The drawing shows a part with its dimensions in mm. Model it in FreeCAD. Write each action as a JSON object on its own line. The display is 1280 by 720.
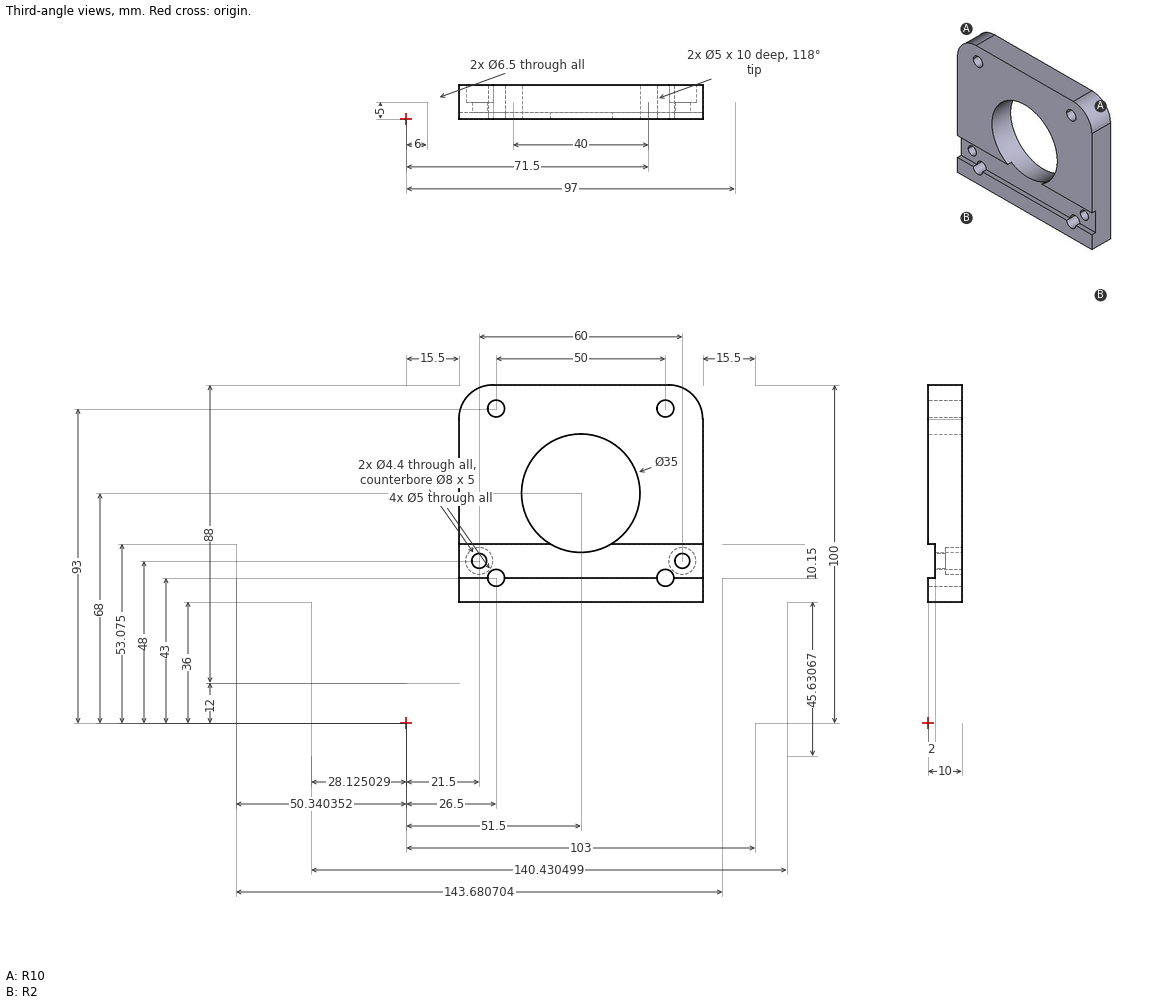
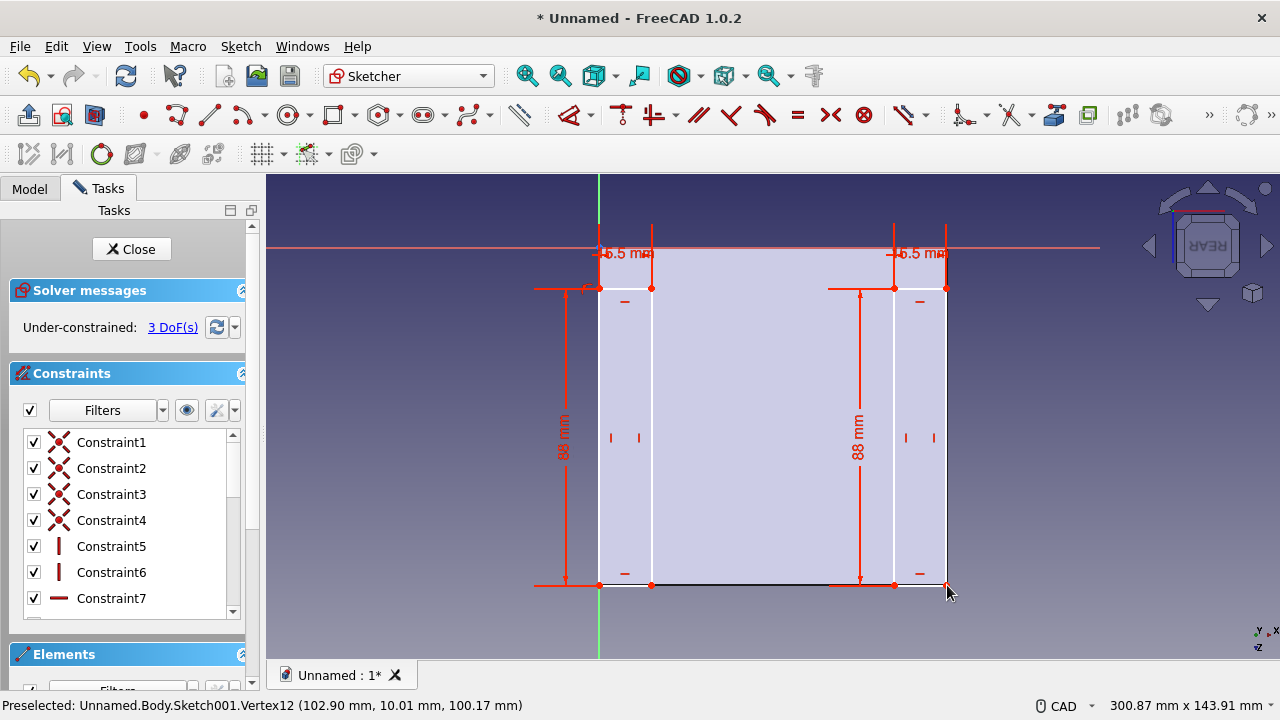
{"action": "left_click", "coordinate": [568, 116]}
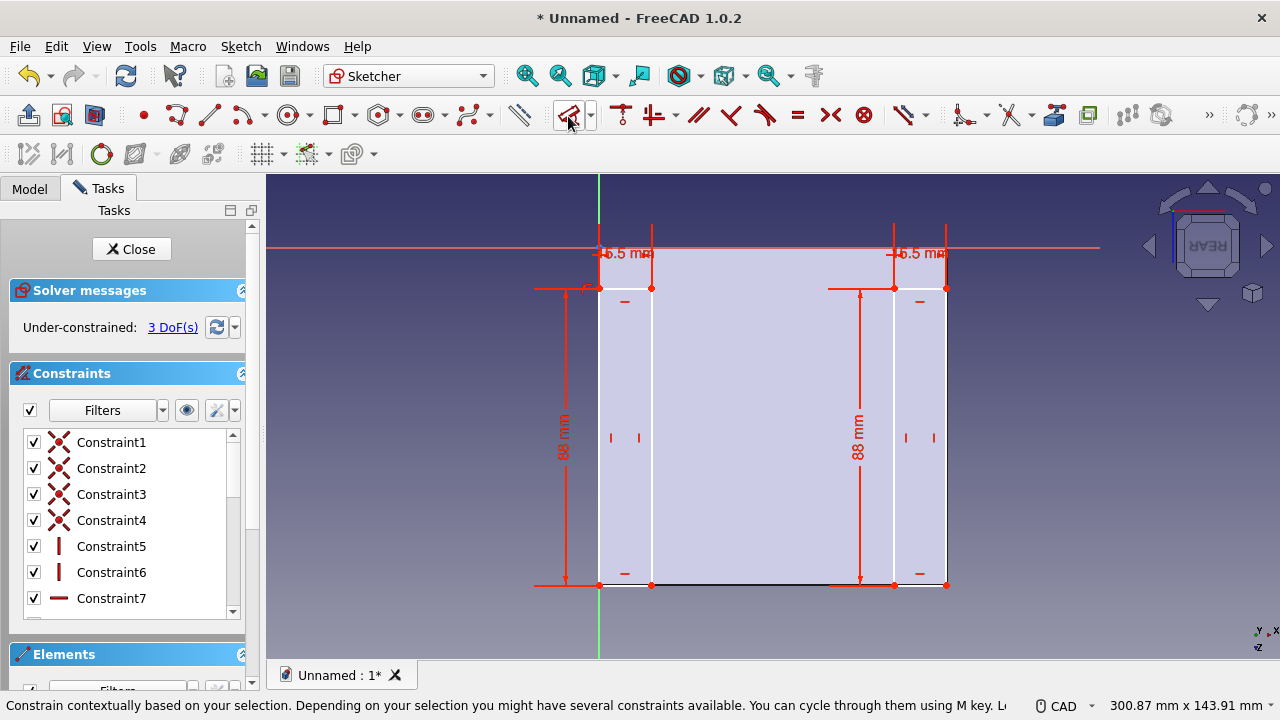
{"action": "left_click", "coordinate": [599, 289]}
{"action": "left_click", "coordinate": [565, 268]}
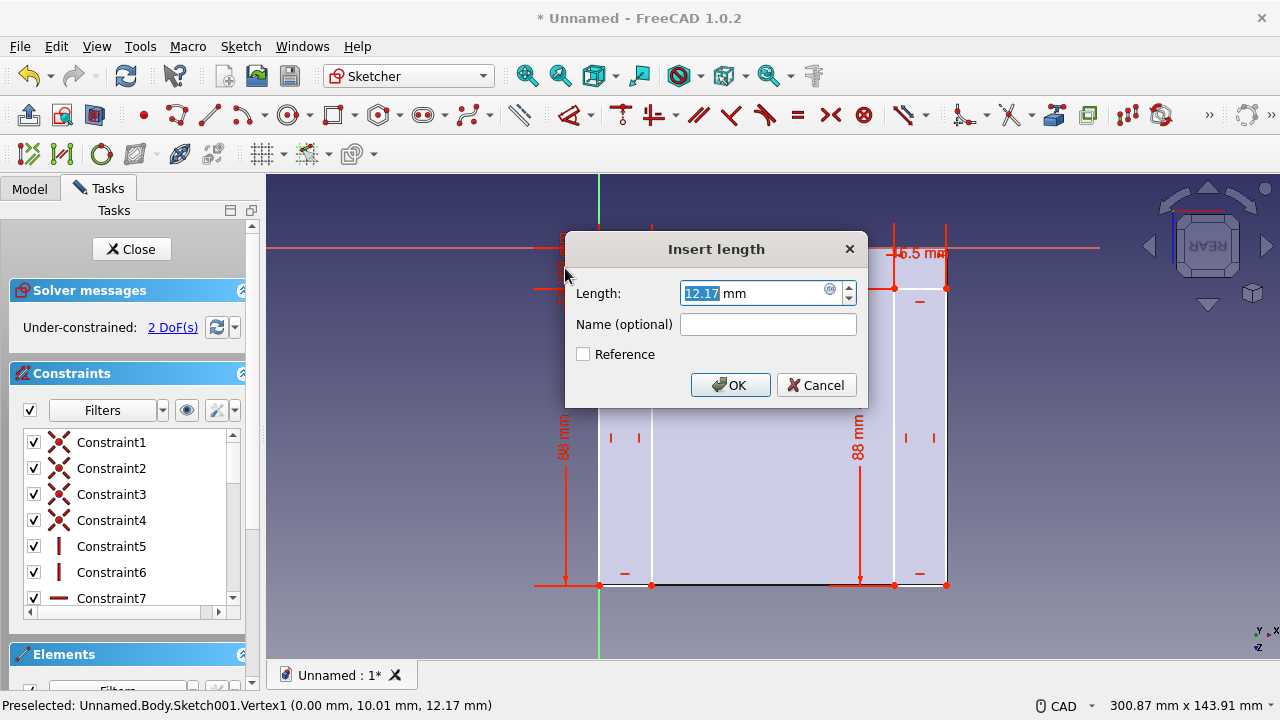
{"action": "type", "text": "12"}
{"action": "key", "text": "Return"}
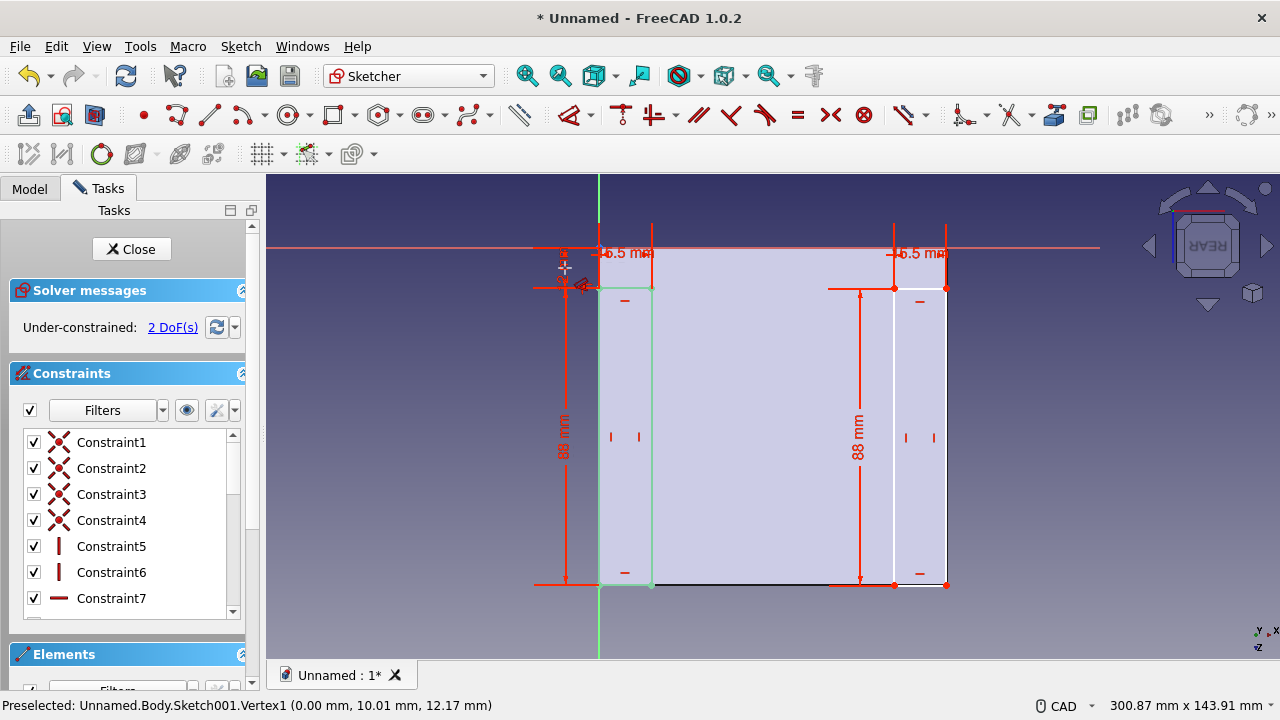
{"action": "left_click", "coordinate": [894, 289]}
{"action": "left_click", "coordinate": [928, 268]}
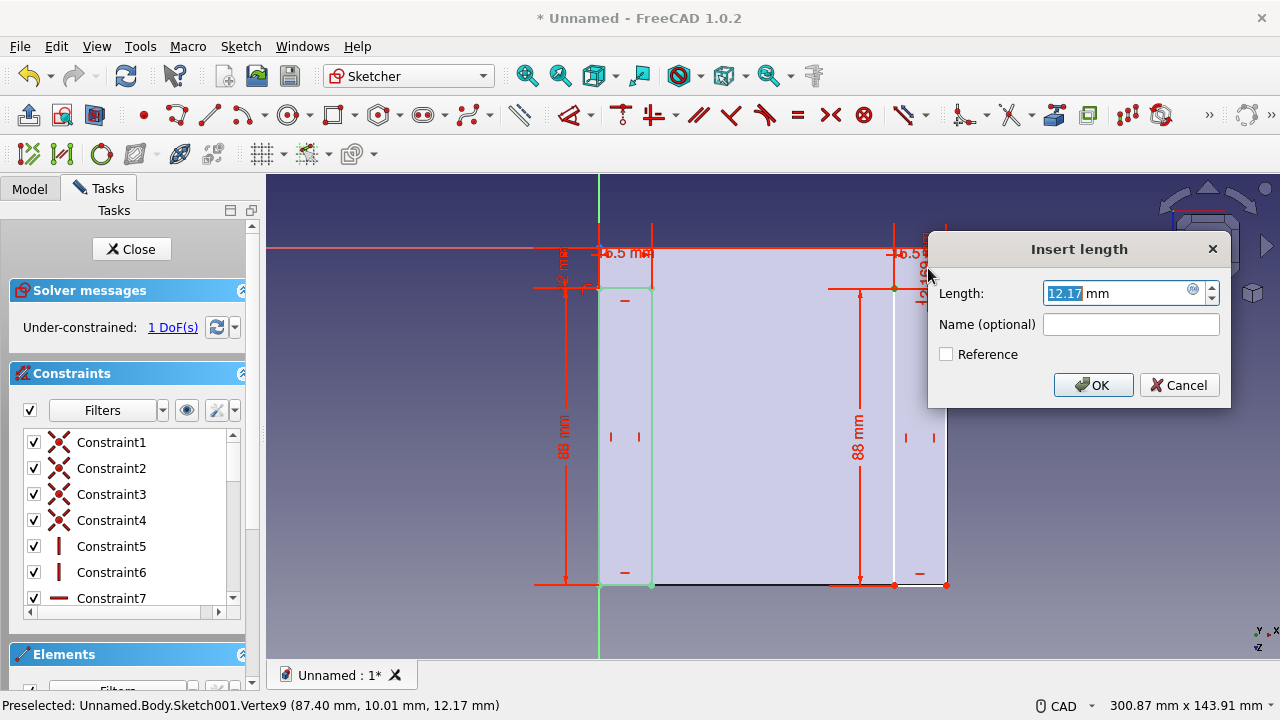
{"action": "type", "text": "12"}
{"action": "key", "text": "Return"}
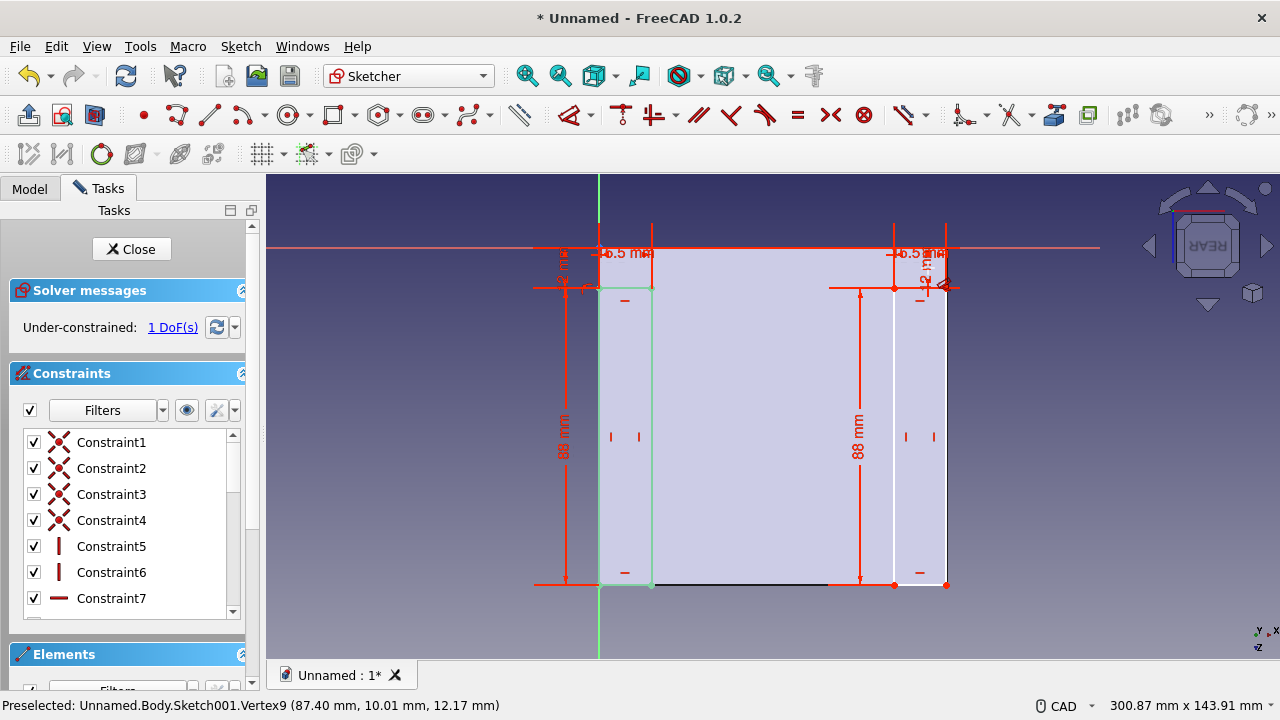
{"action": "left_click", "coordinate": [946, 585]}
{"action": "left_click", "coordinate": [773, 619]}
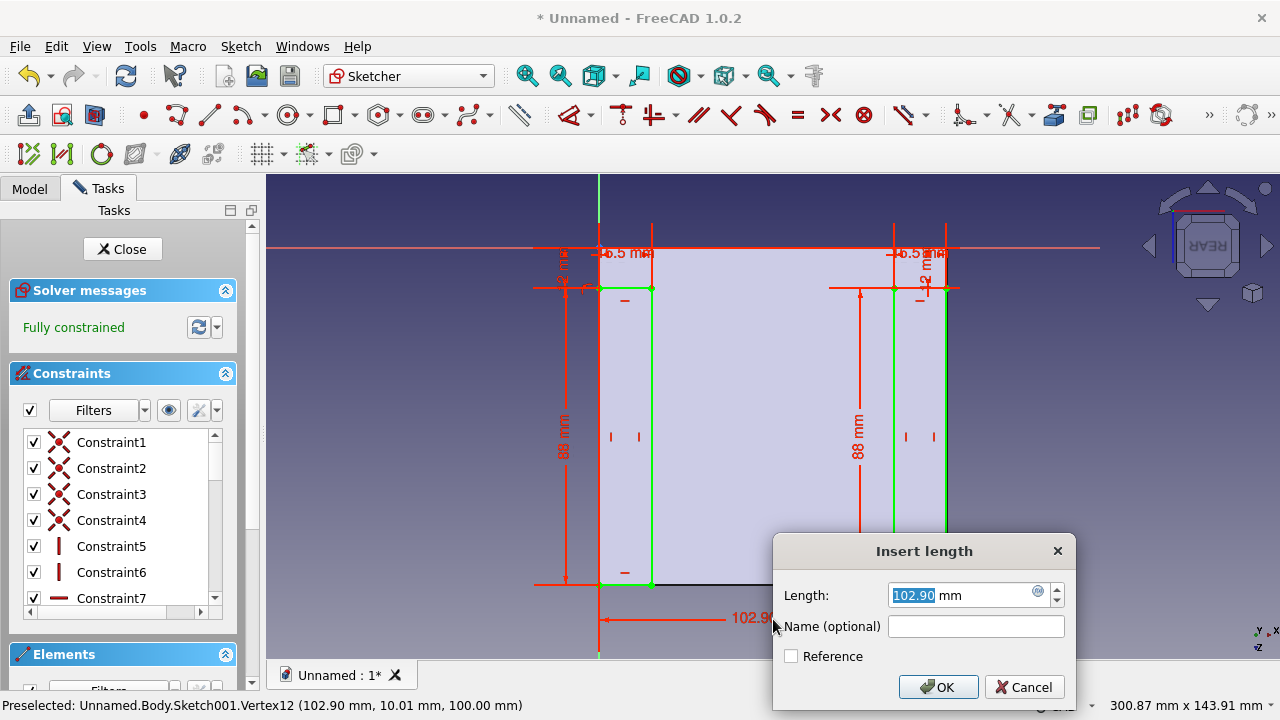
{"action": "type", "text": "103"}
{"action": "key", "text": "Return"}
{"action": "key", "text": "Escape"}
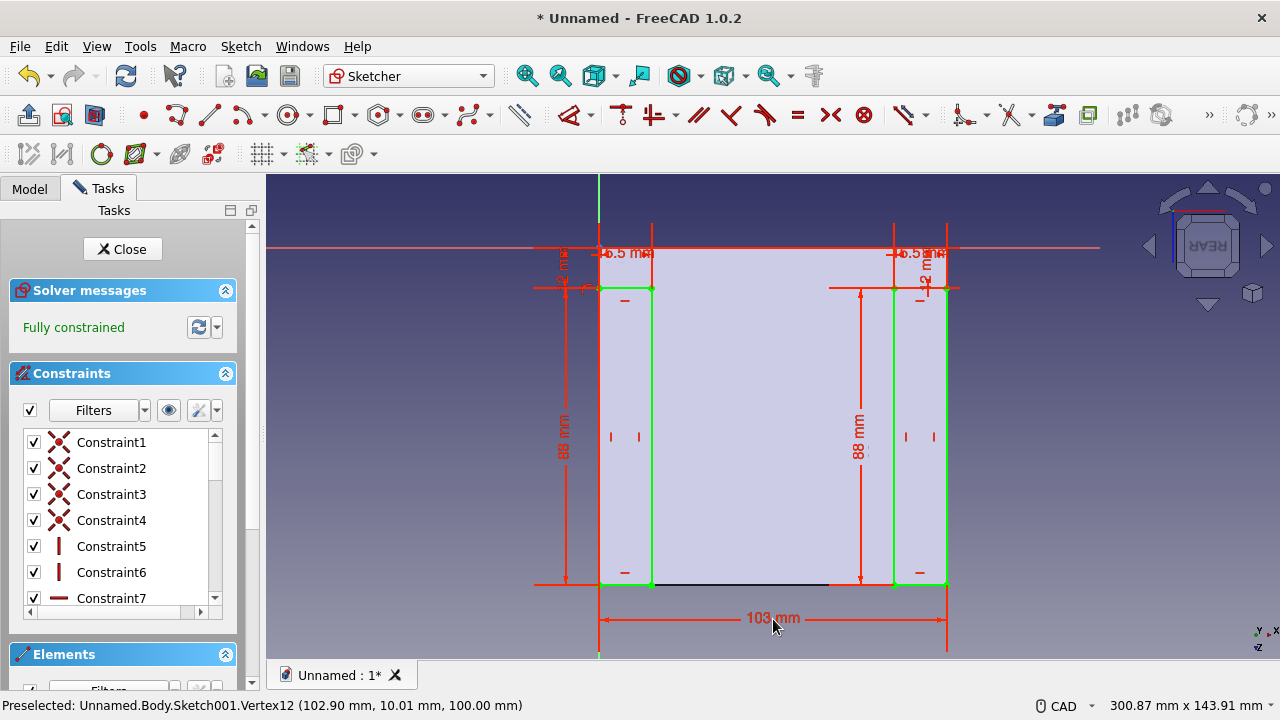
{"action": "left_click", "coordinate": [123, 249]}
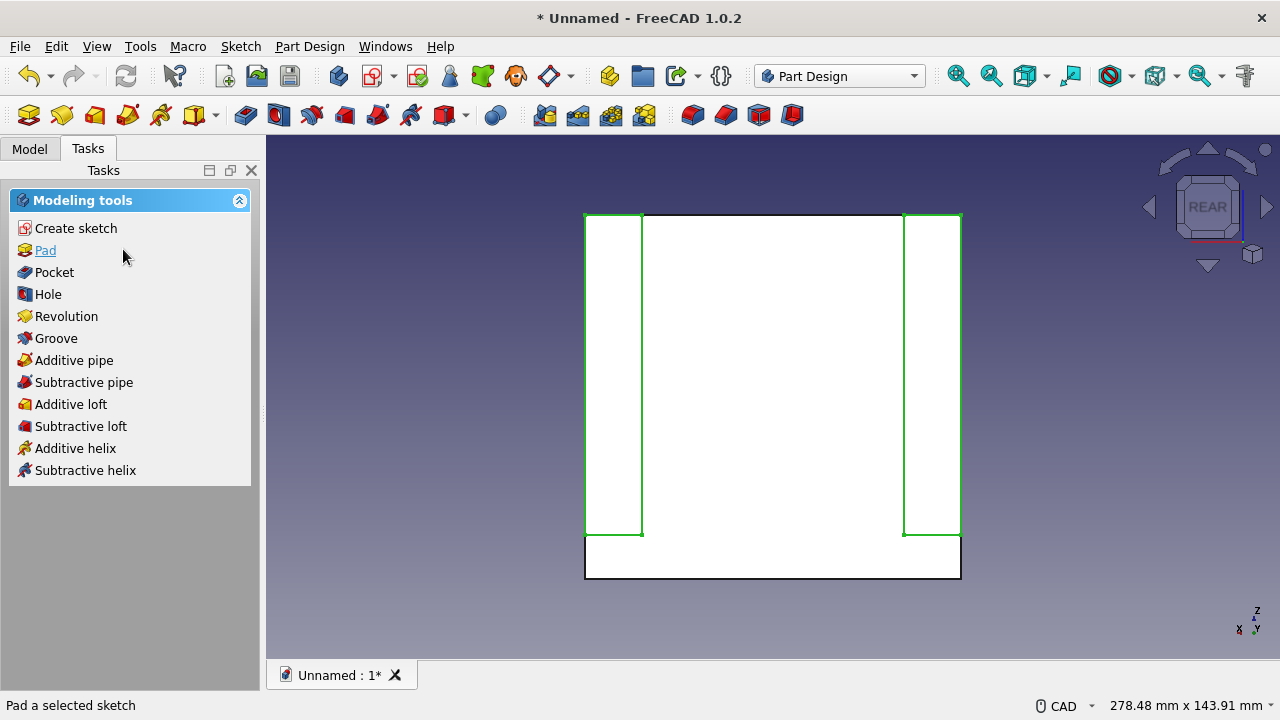
{"action": "left_click", "coordinate": [246, 116]}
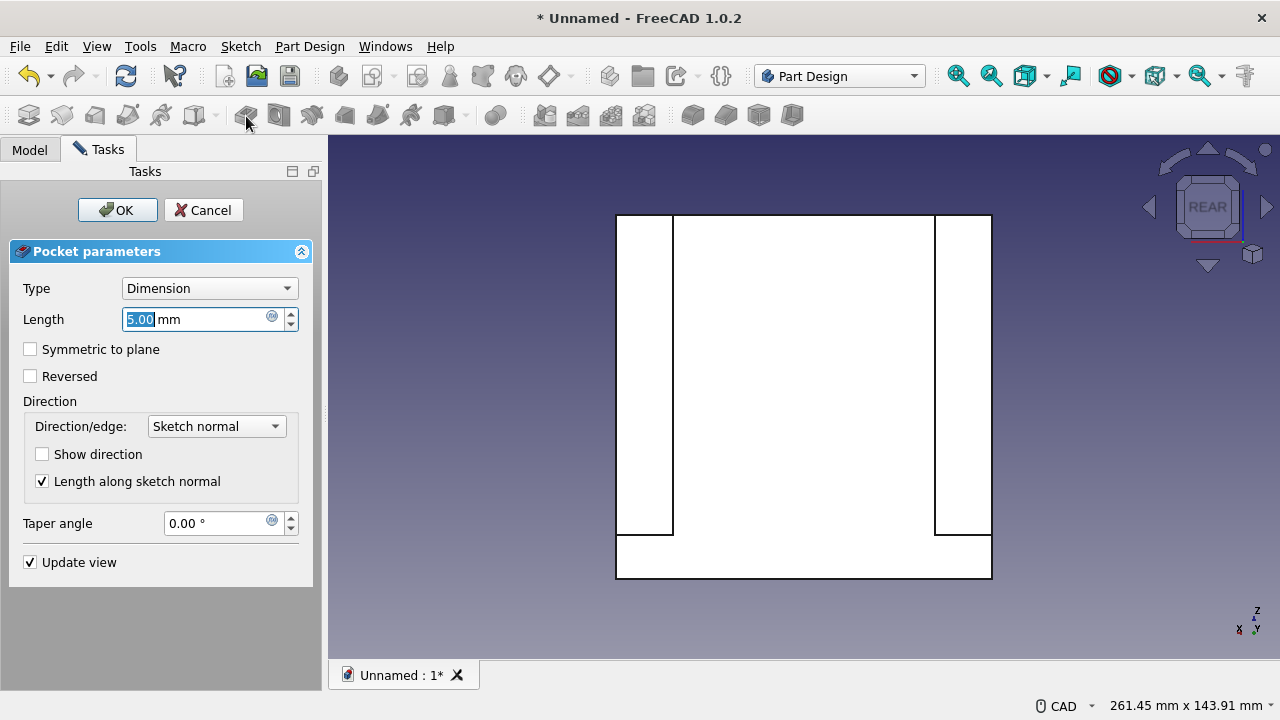
{"action": "left_click", "coordinate": [210, 288]}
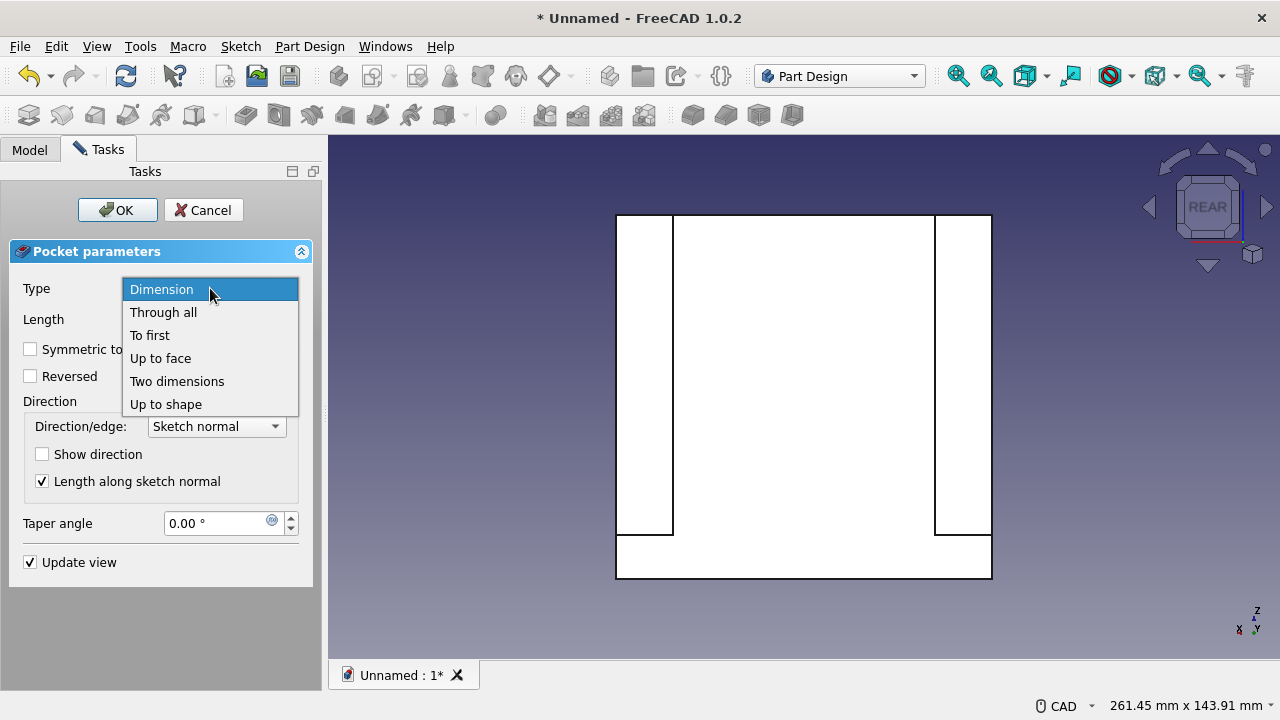
{"action": "left_click", "coordinate": [208, 312]}